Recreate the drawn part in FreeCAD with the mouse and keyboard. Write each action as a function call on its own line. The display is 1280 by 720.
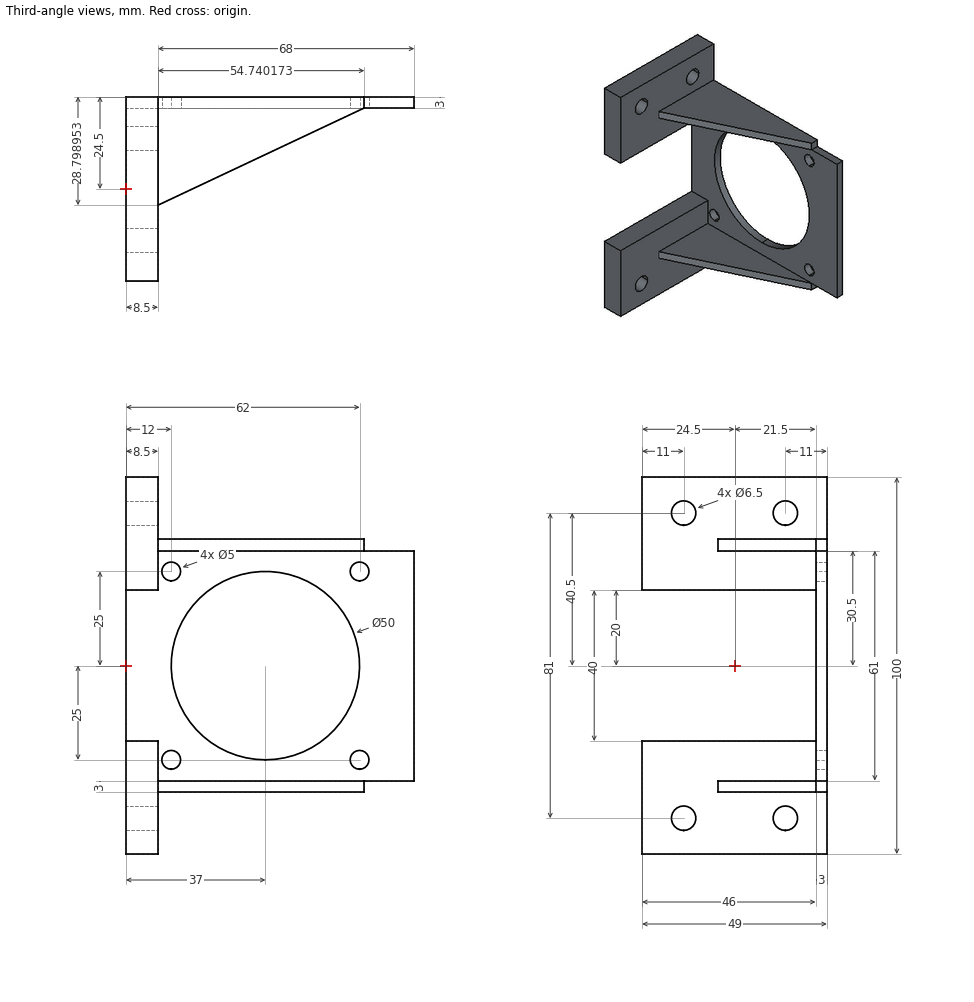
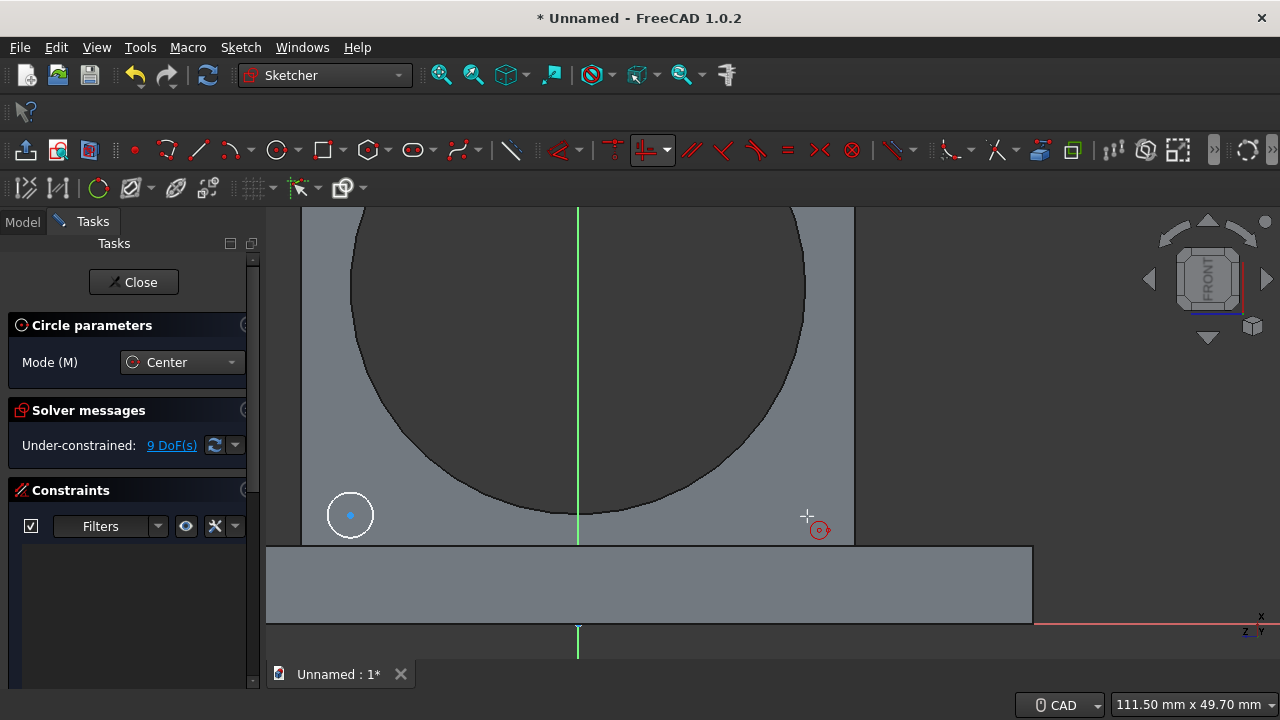
click(805, 514)
click(821, 498)
key(Escape)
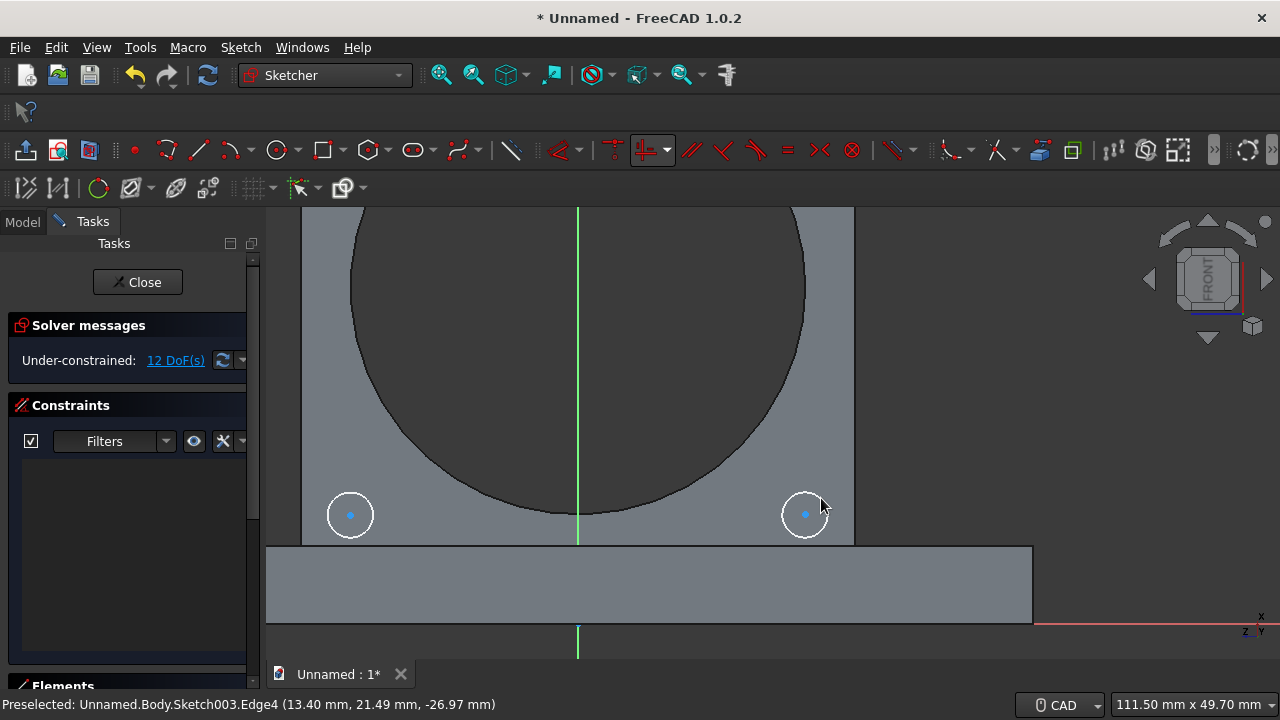
click(366, 499)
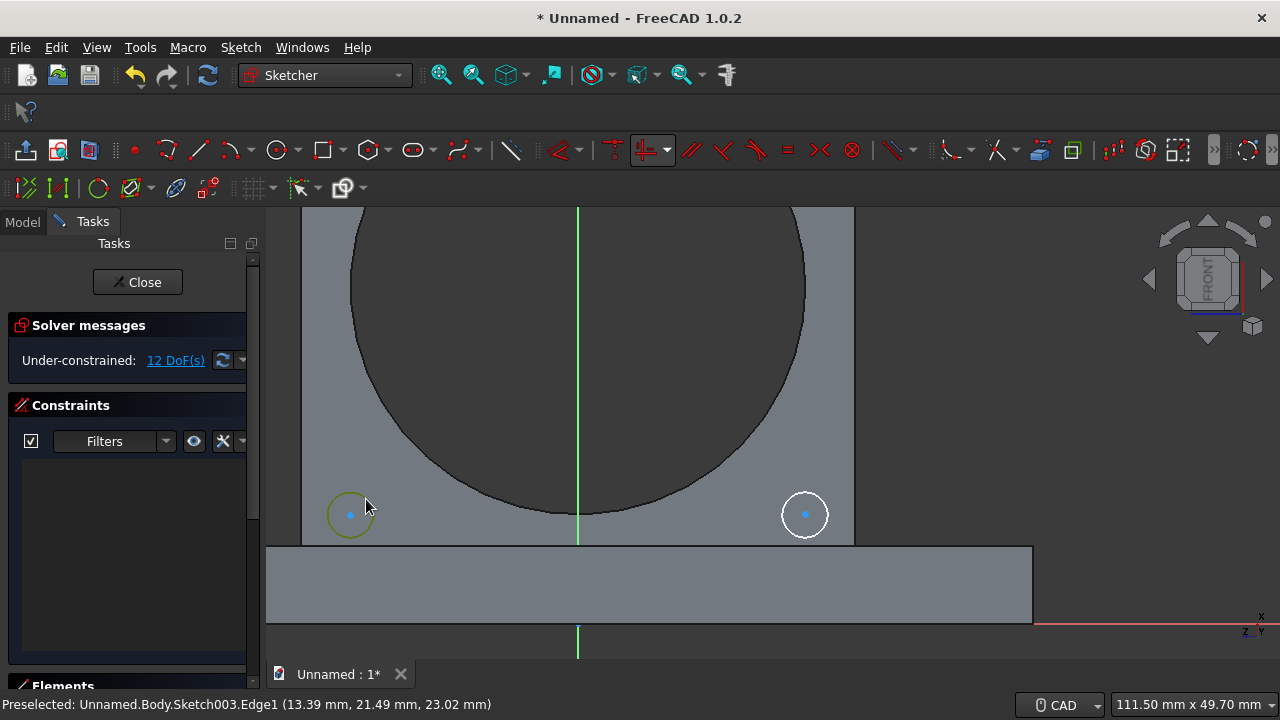
scroll(808, 517, down, 4)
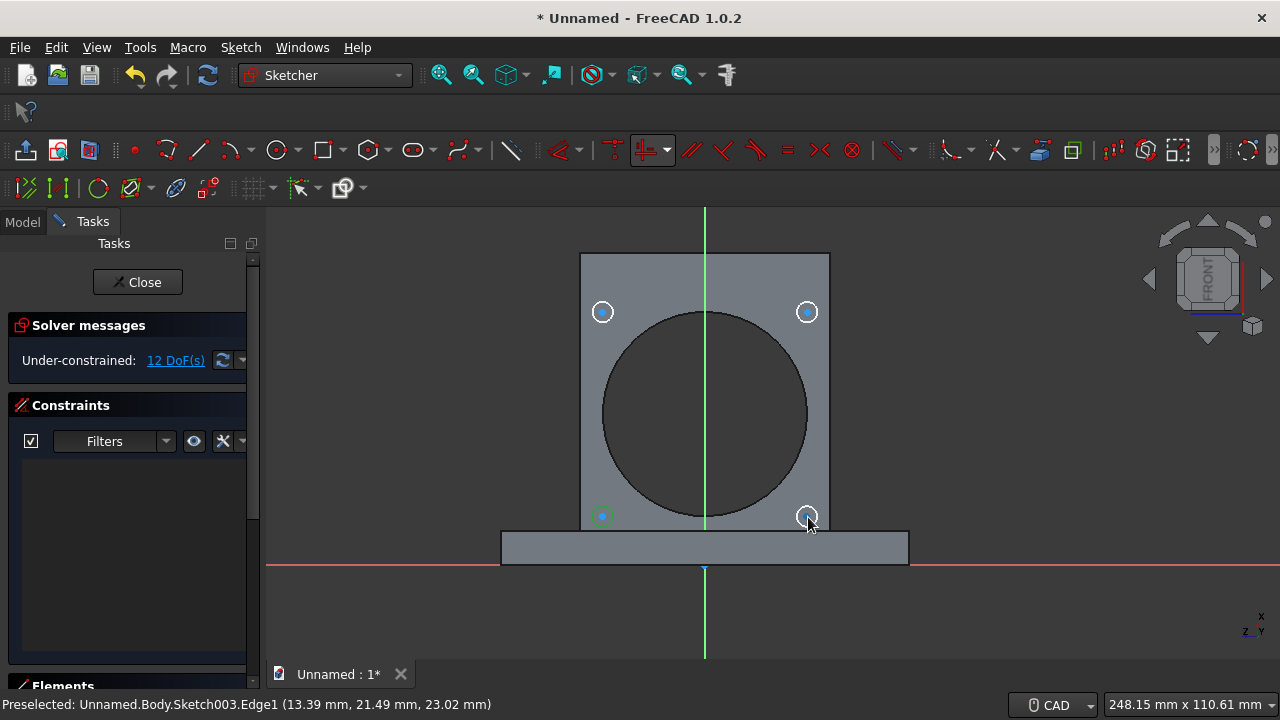
scroll(610, 305, up, 2)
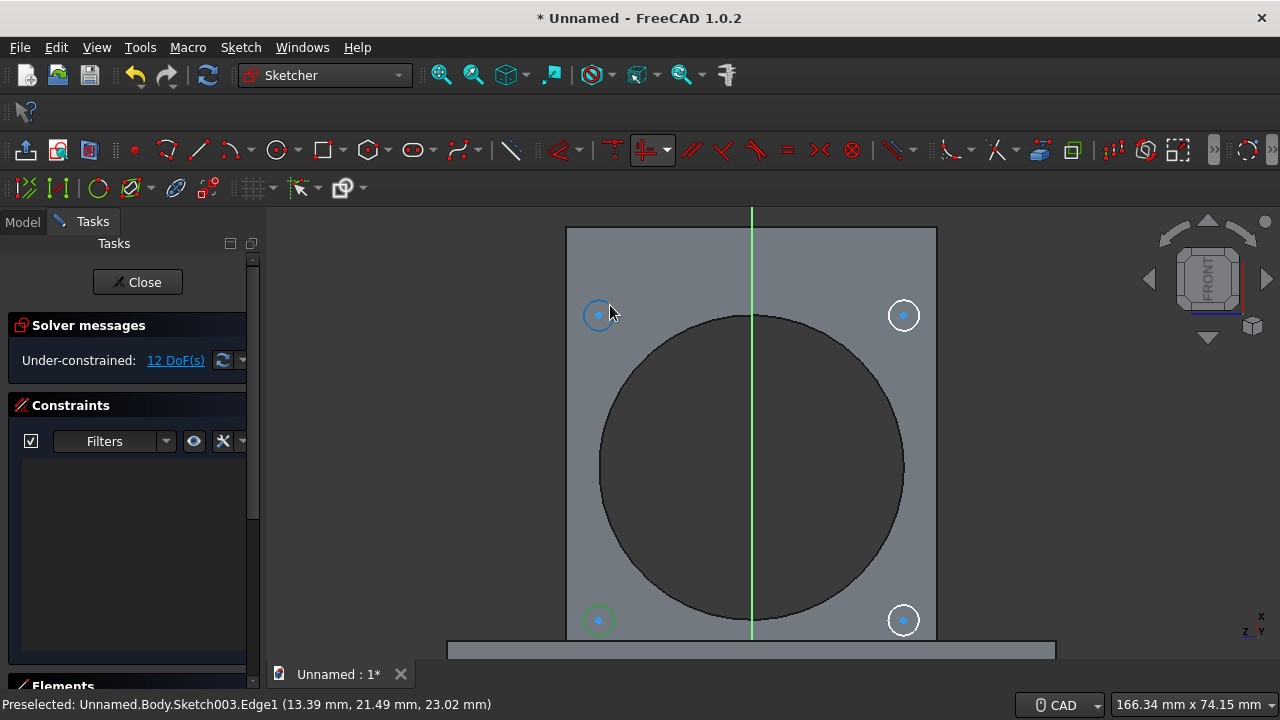
click(610, 305)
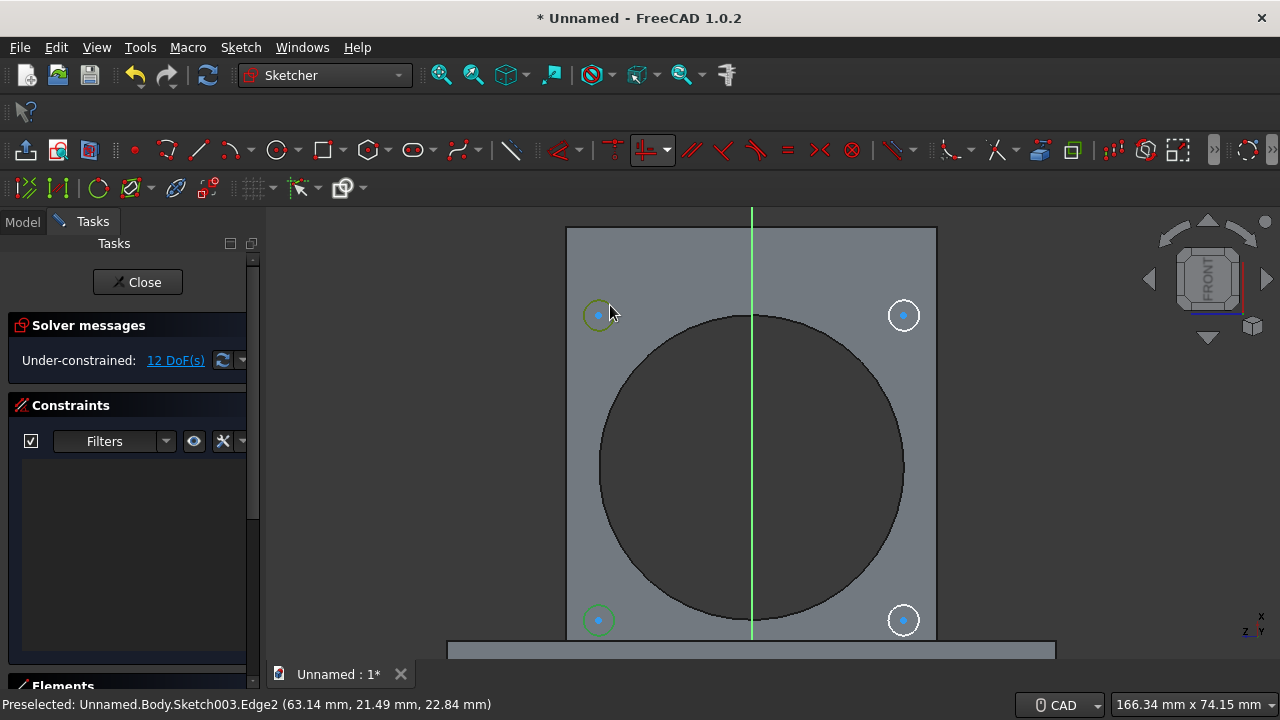
click(915, 305)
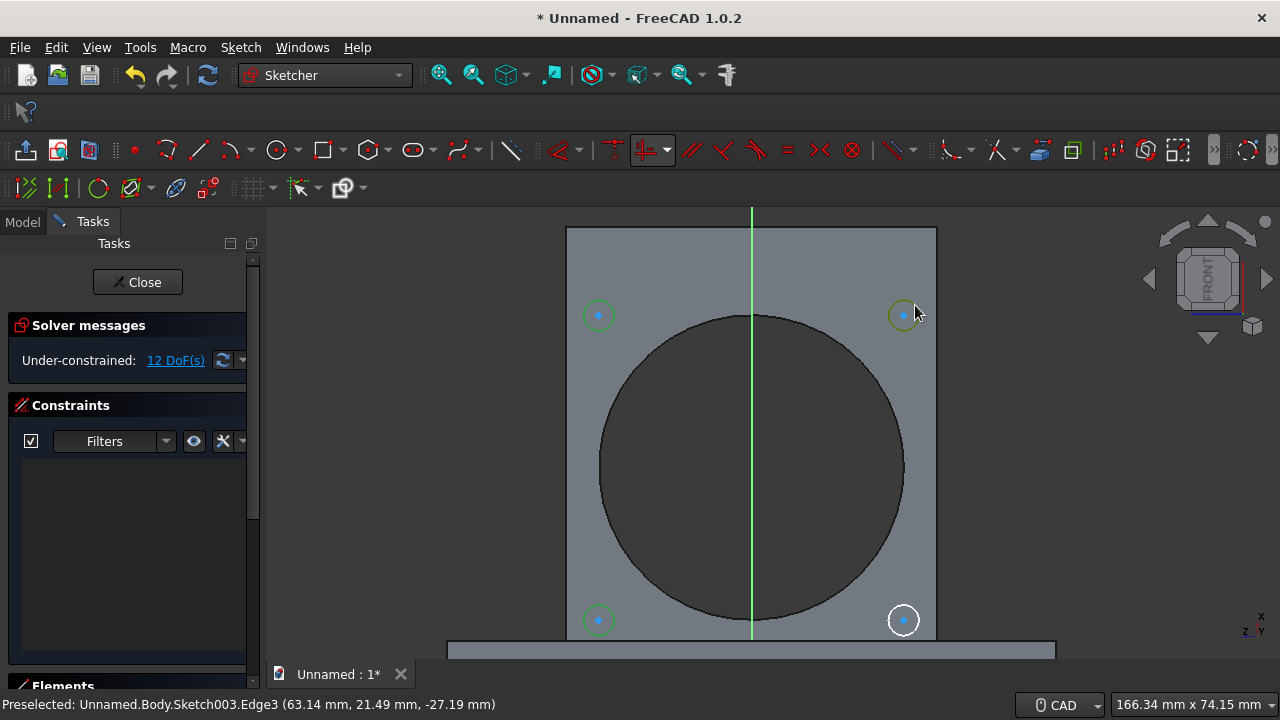
click(914, 610)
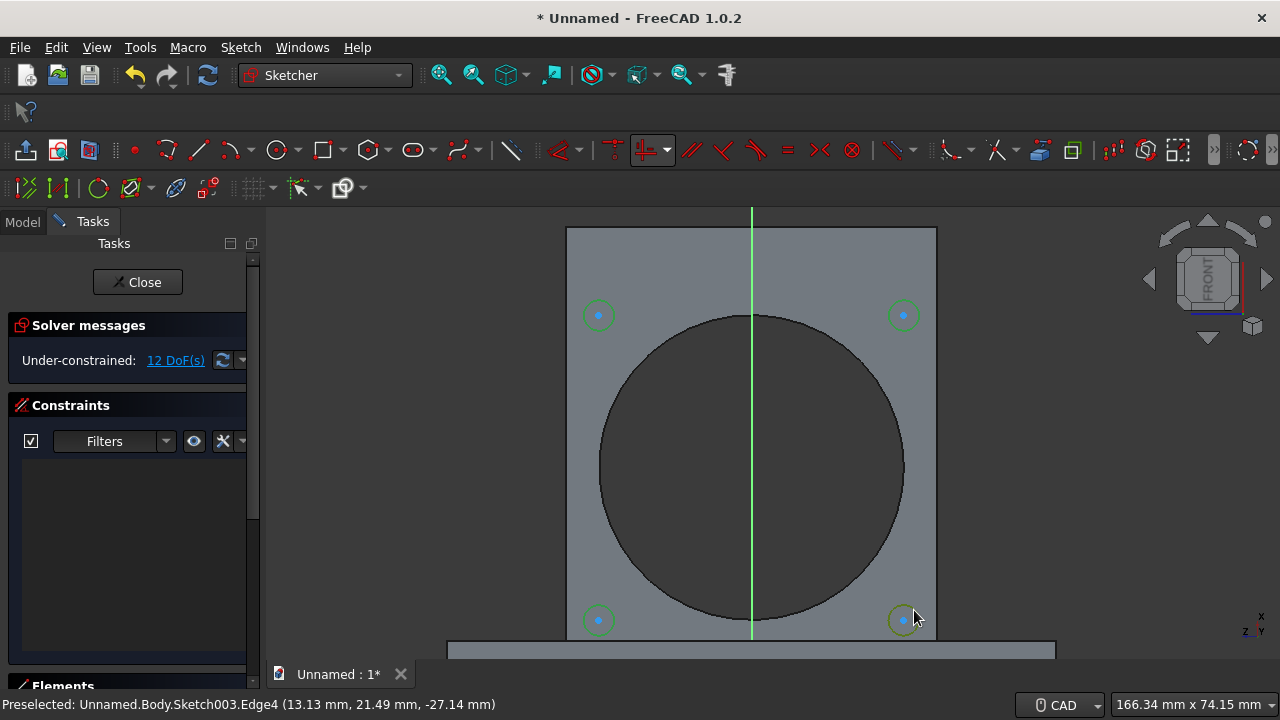
click(788, 150)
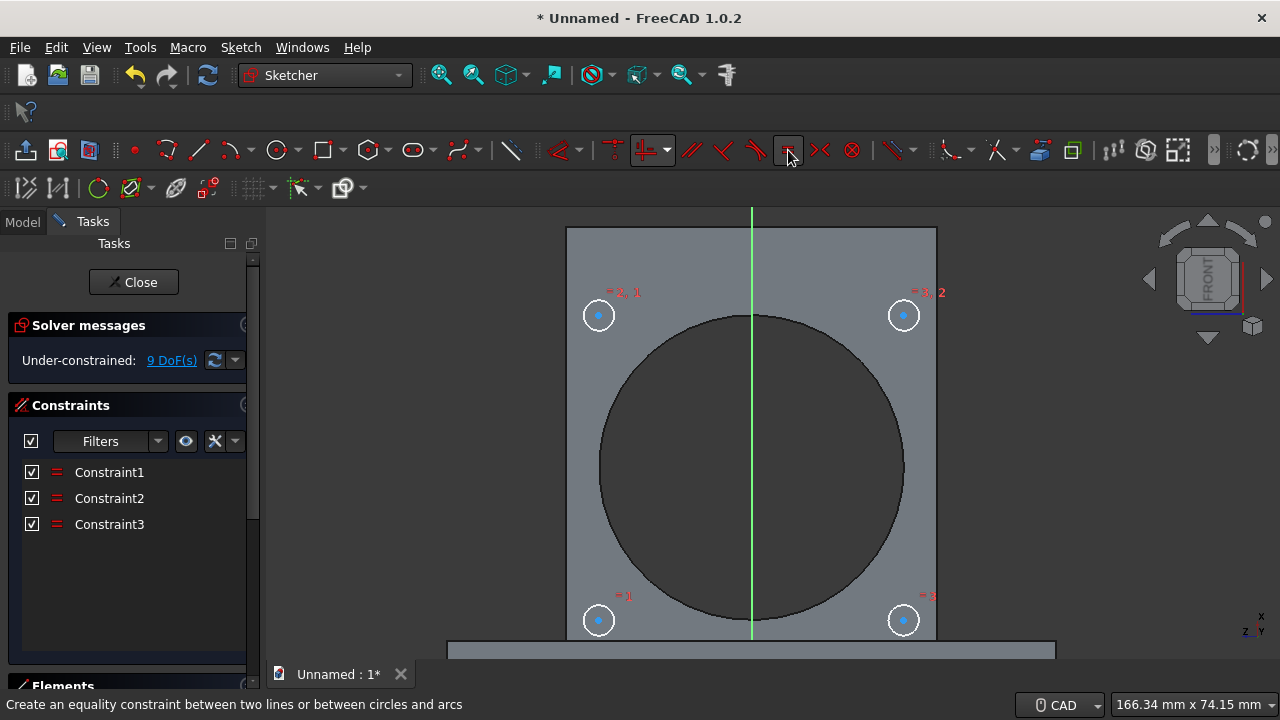
click(599, 620)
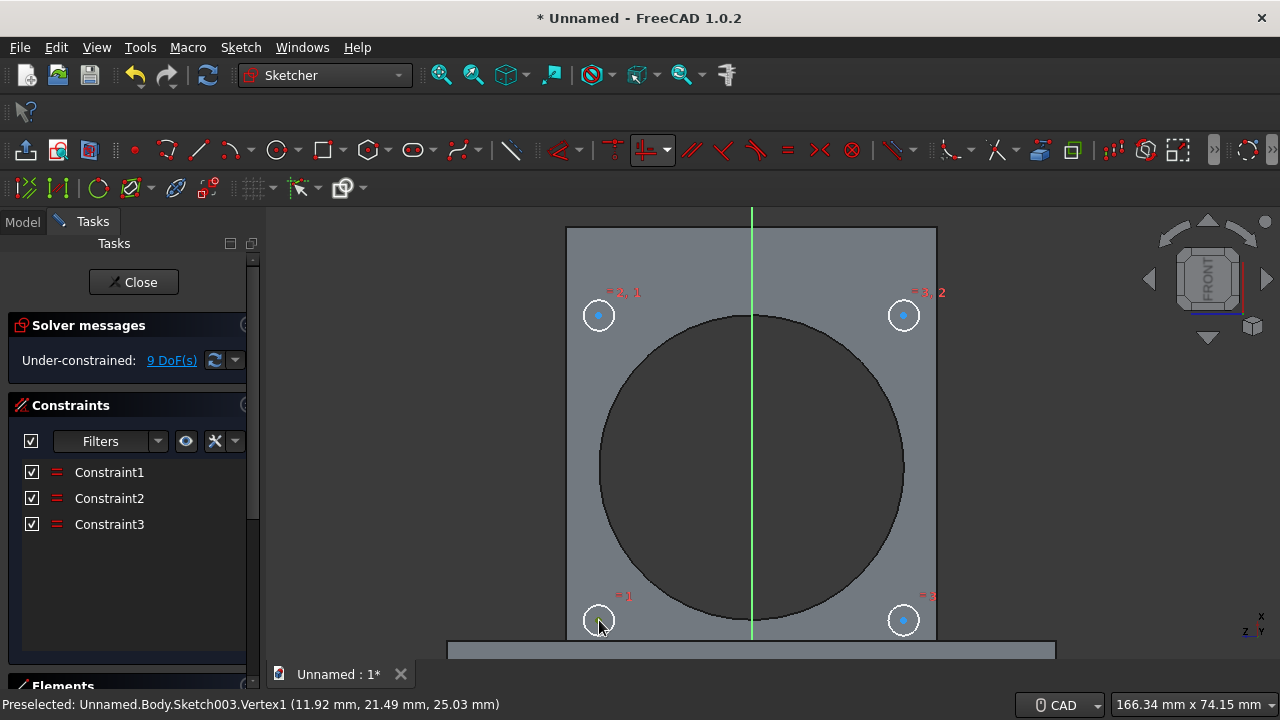
click(599, 316)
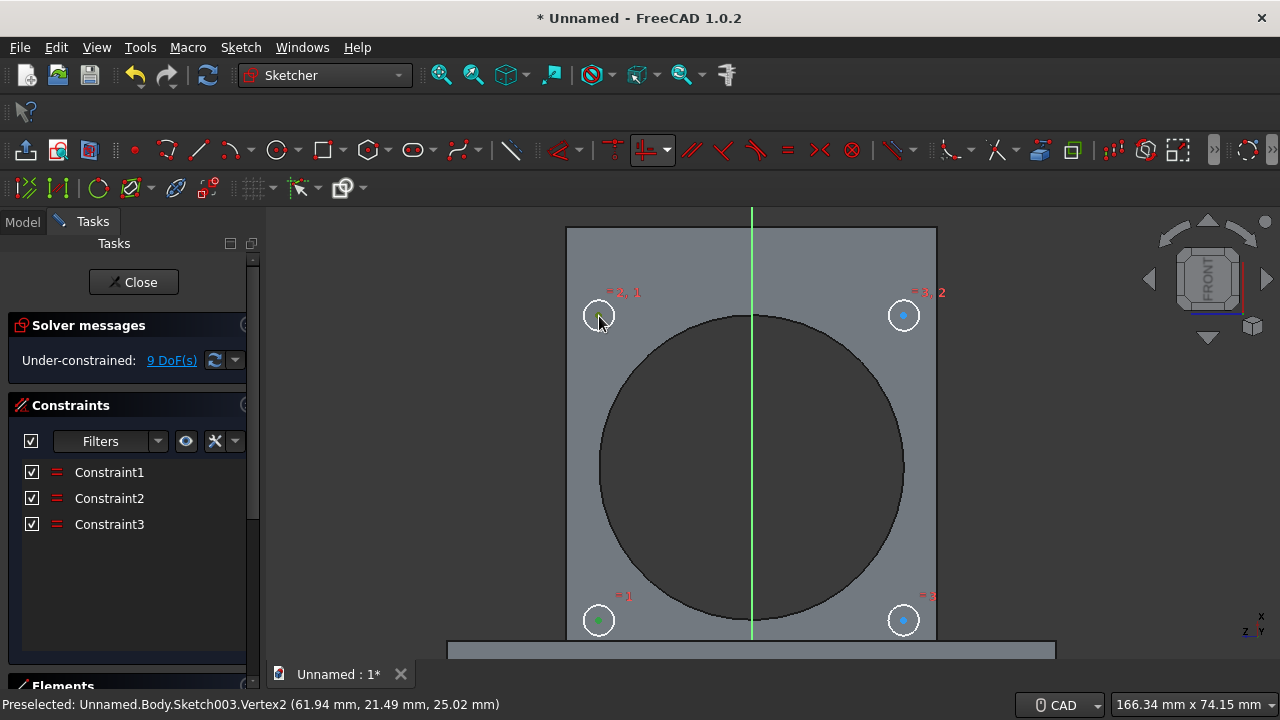
key(v)